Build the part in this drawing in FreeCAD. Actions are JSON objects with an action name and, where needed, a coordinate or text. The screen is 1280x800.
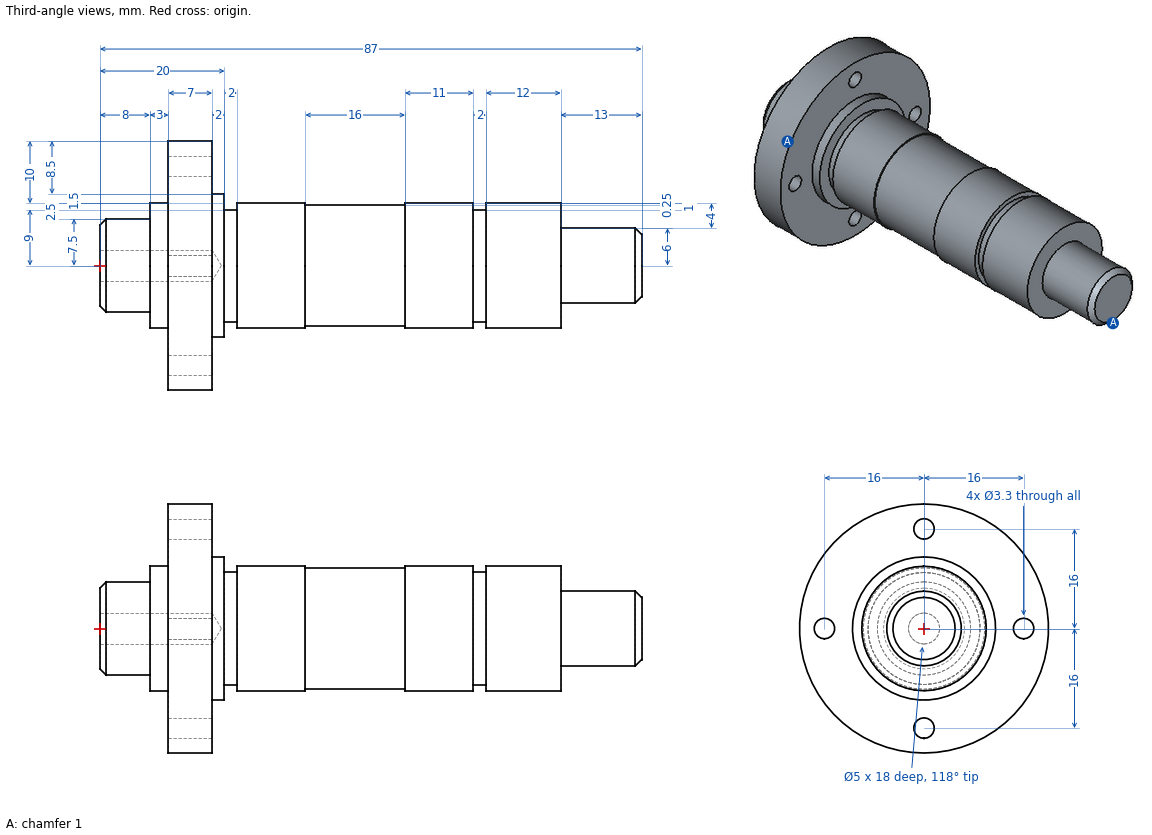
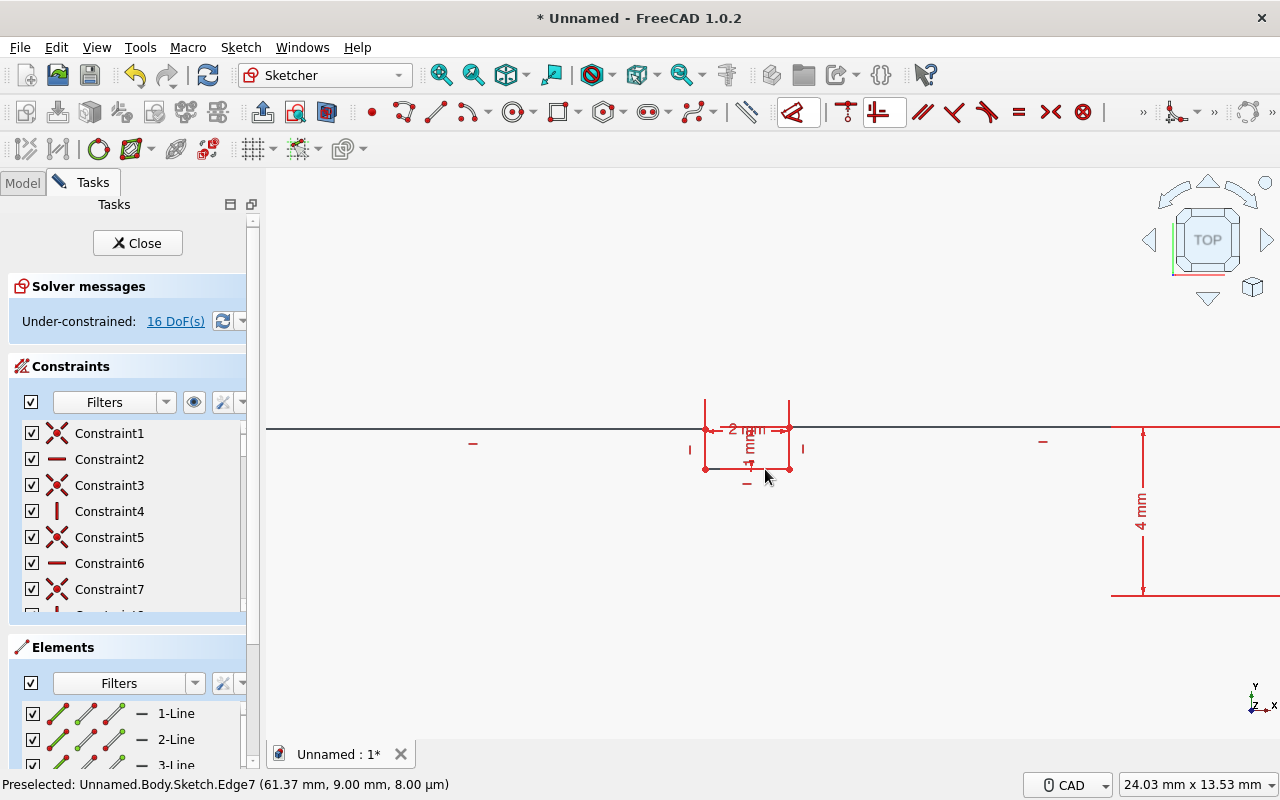
{"action": "left_click", "coordinate": [705, 457]}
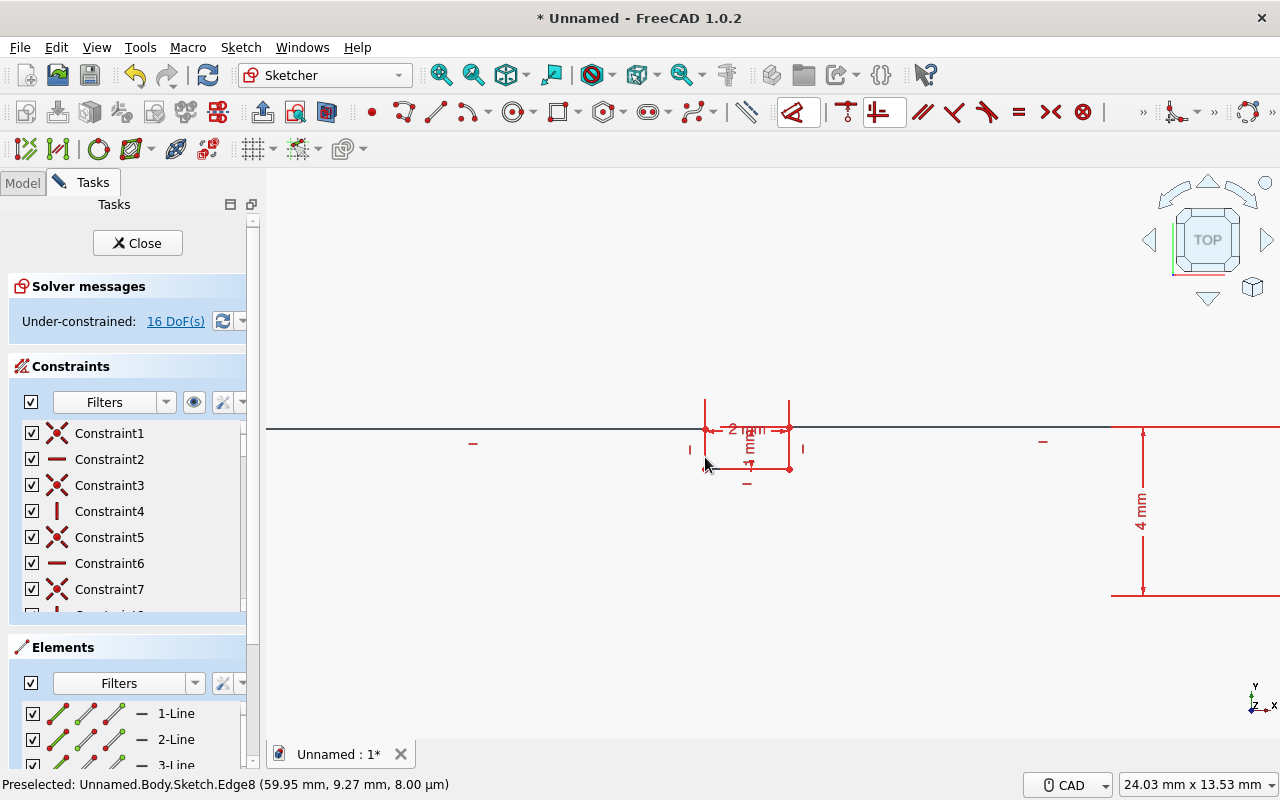
{"action": "left_click", "coordinate": [814, 112]}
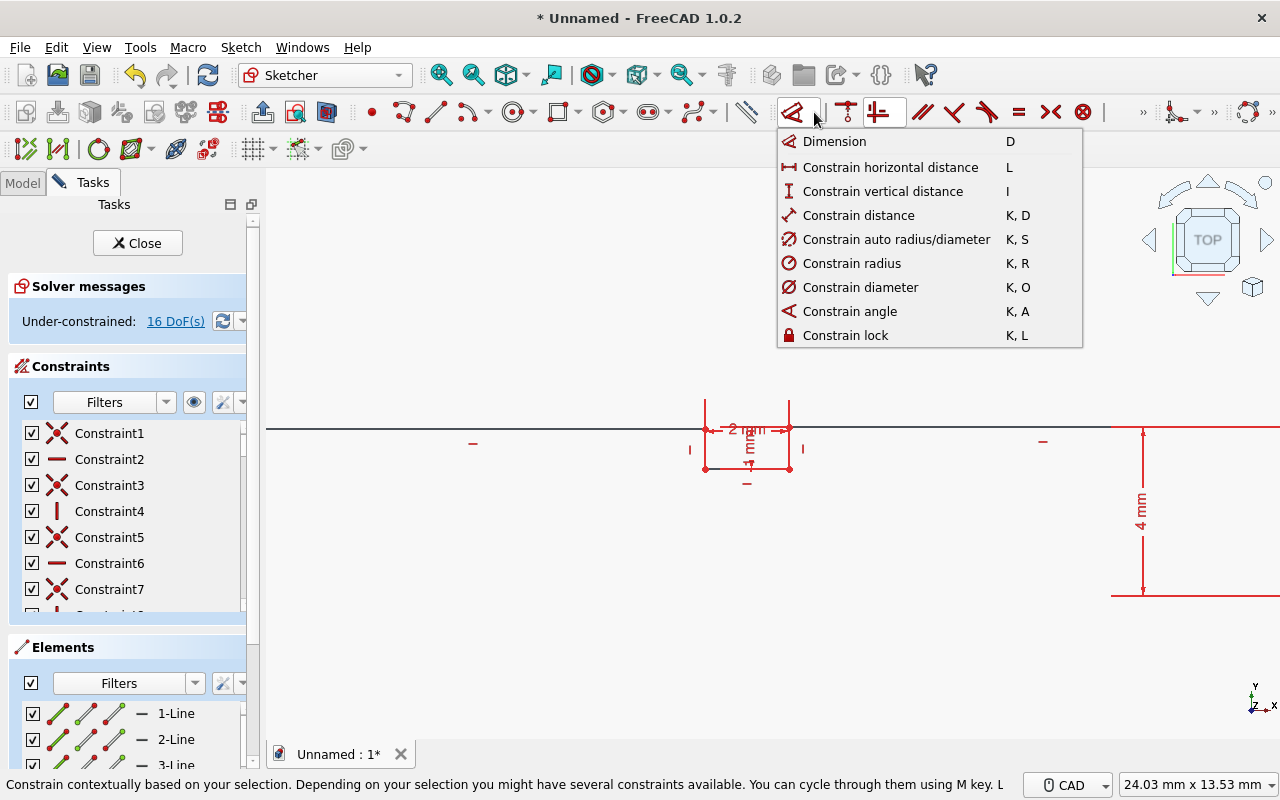
{"action": "left_click", "coordinate": [930, 191]}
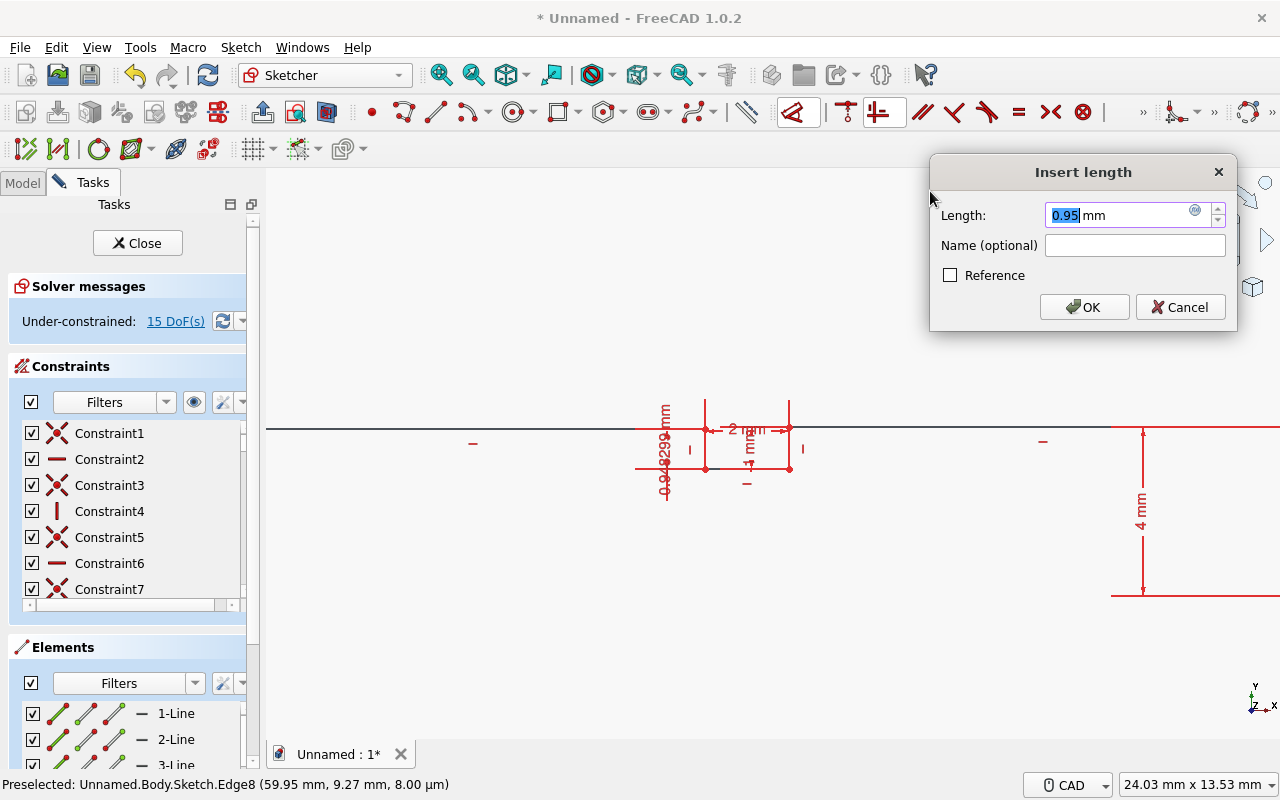
{"action": "type", "text": "1"}
{"action": "key", "text": "Return"}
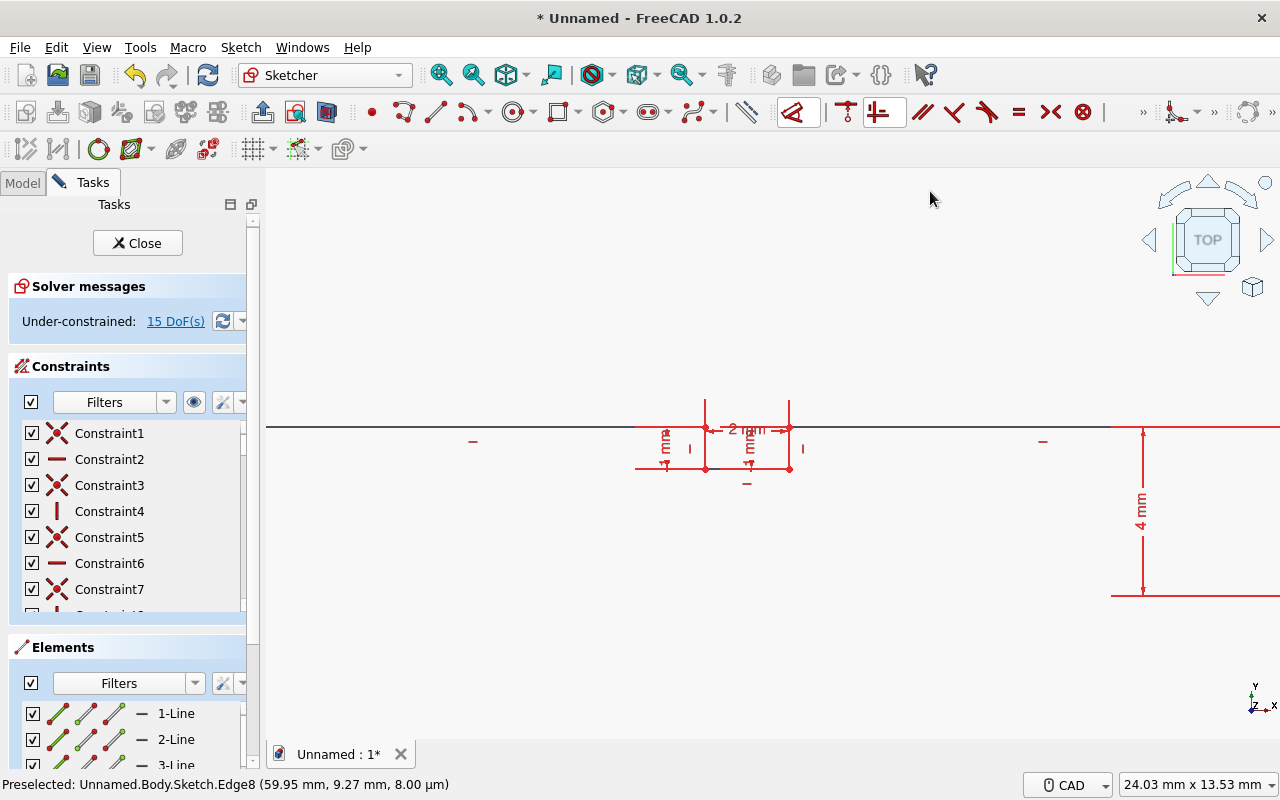
{"action": "scroll", "coordinate": [842, 459], "scroll_direction": "down", "scroll_amount": 9}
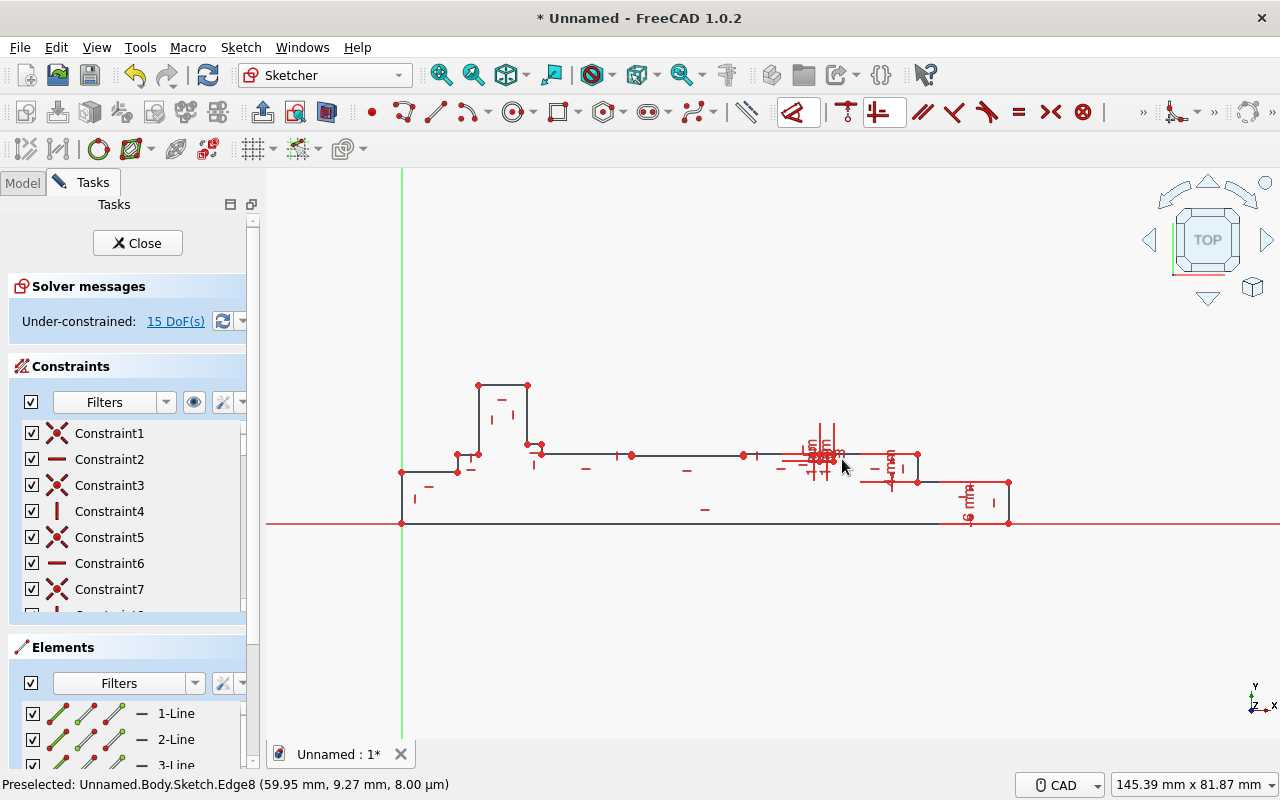
{"action": "scroll", "coordinate": [537, 444], "scroll_direction": "up", "scroll_amount": 6}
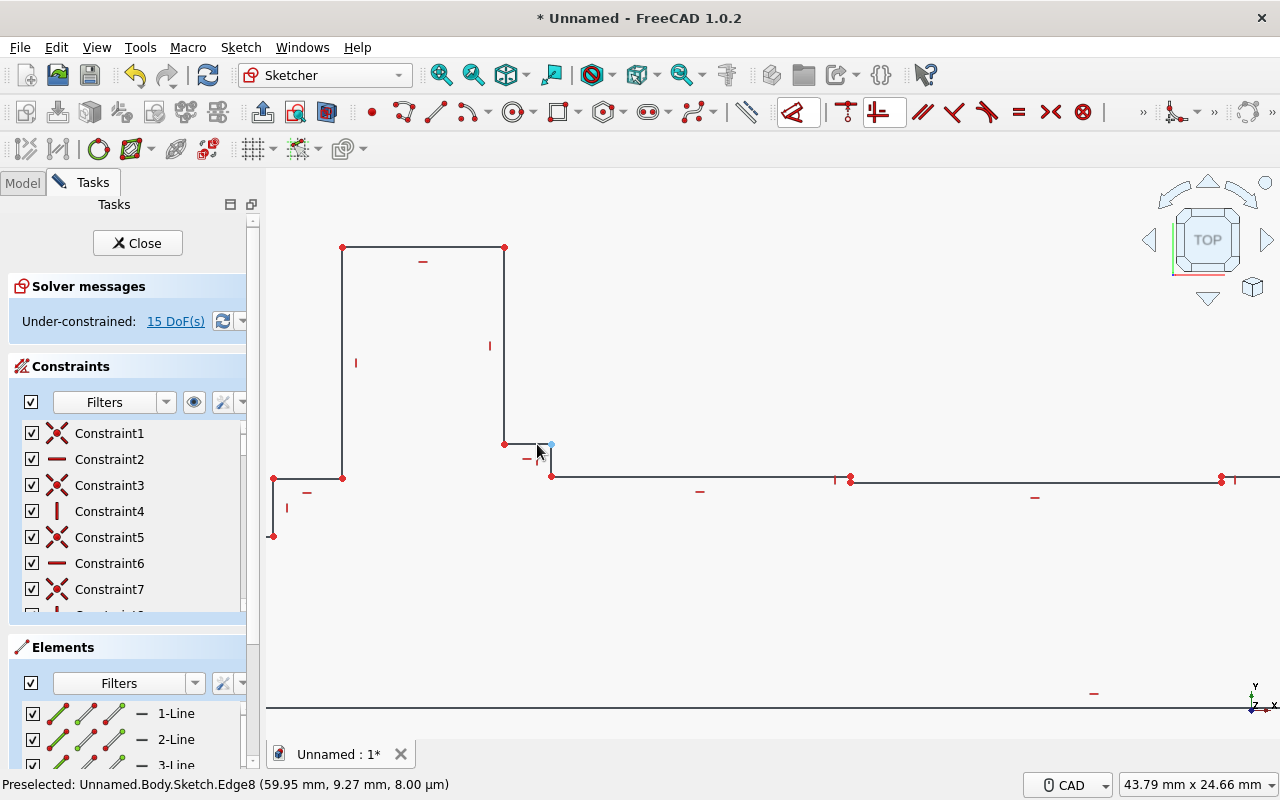
{"action": "left_click", "coordinate": [537, 444]}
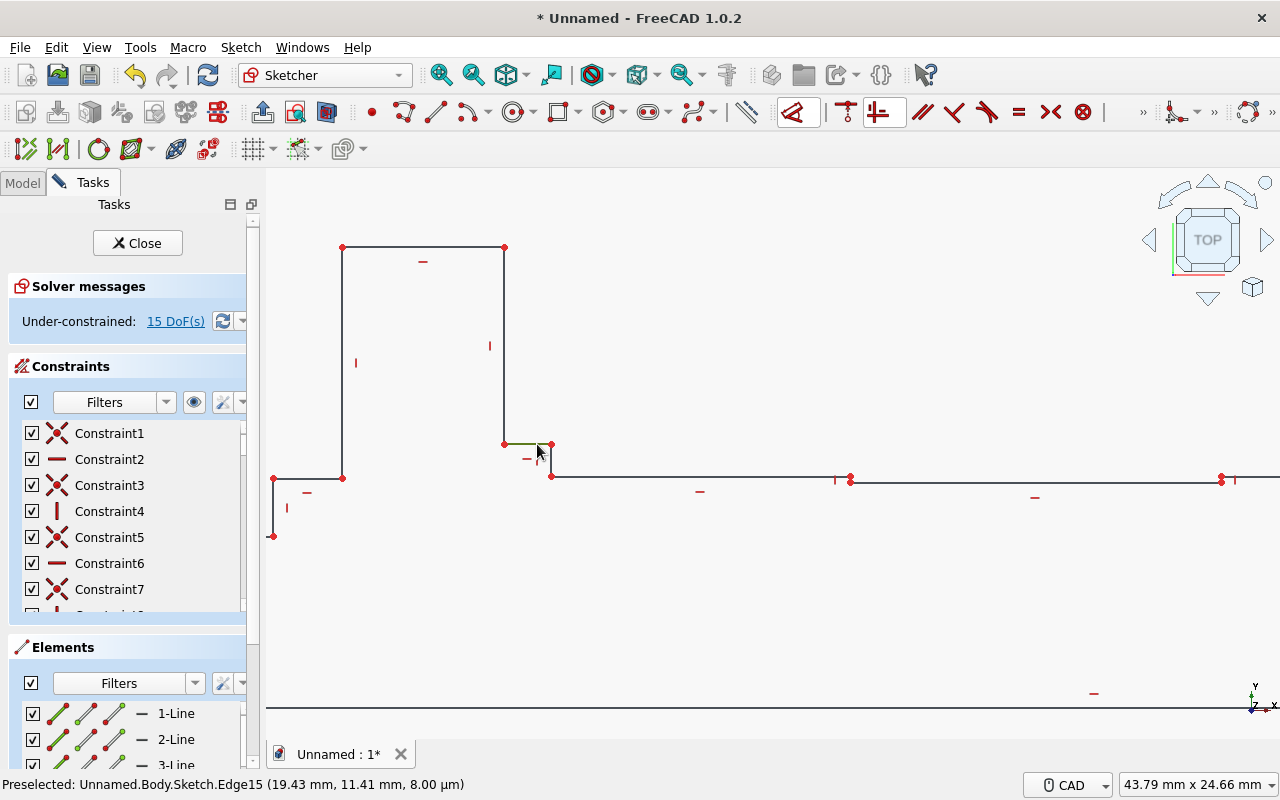
{"action": "key", "text": "l"}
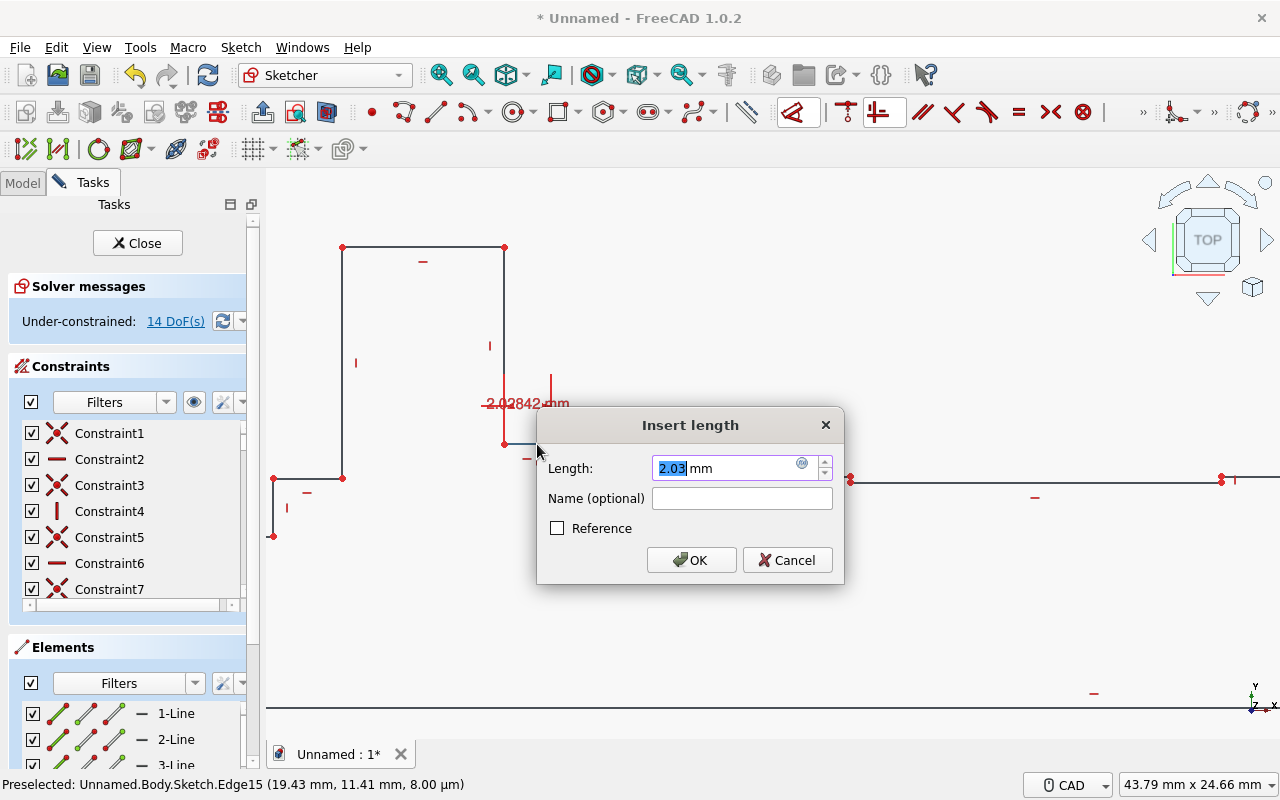
{"action": "type", "text": "2"}
{"action": "key", "text": "Return"}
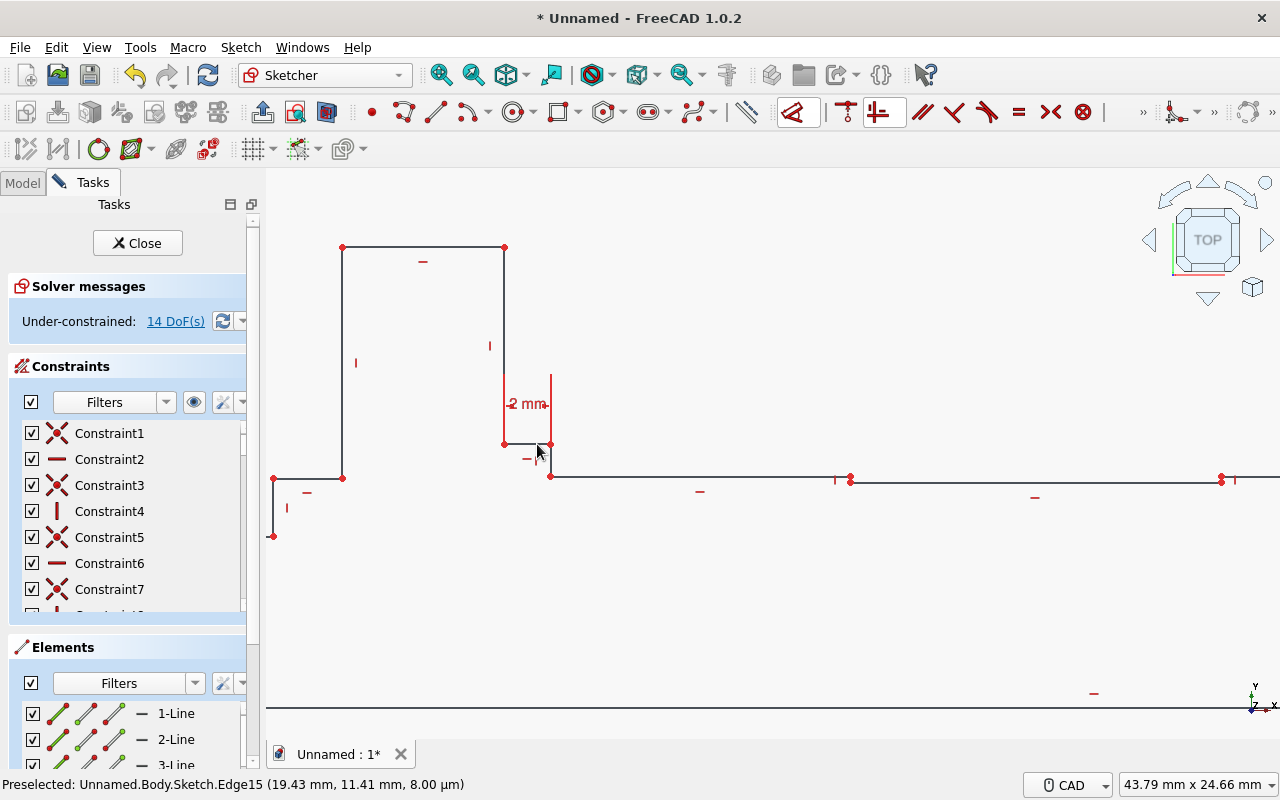
{"action": "left_click", "coordinate": [456, 247]}